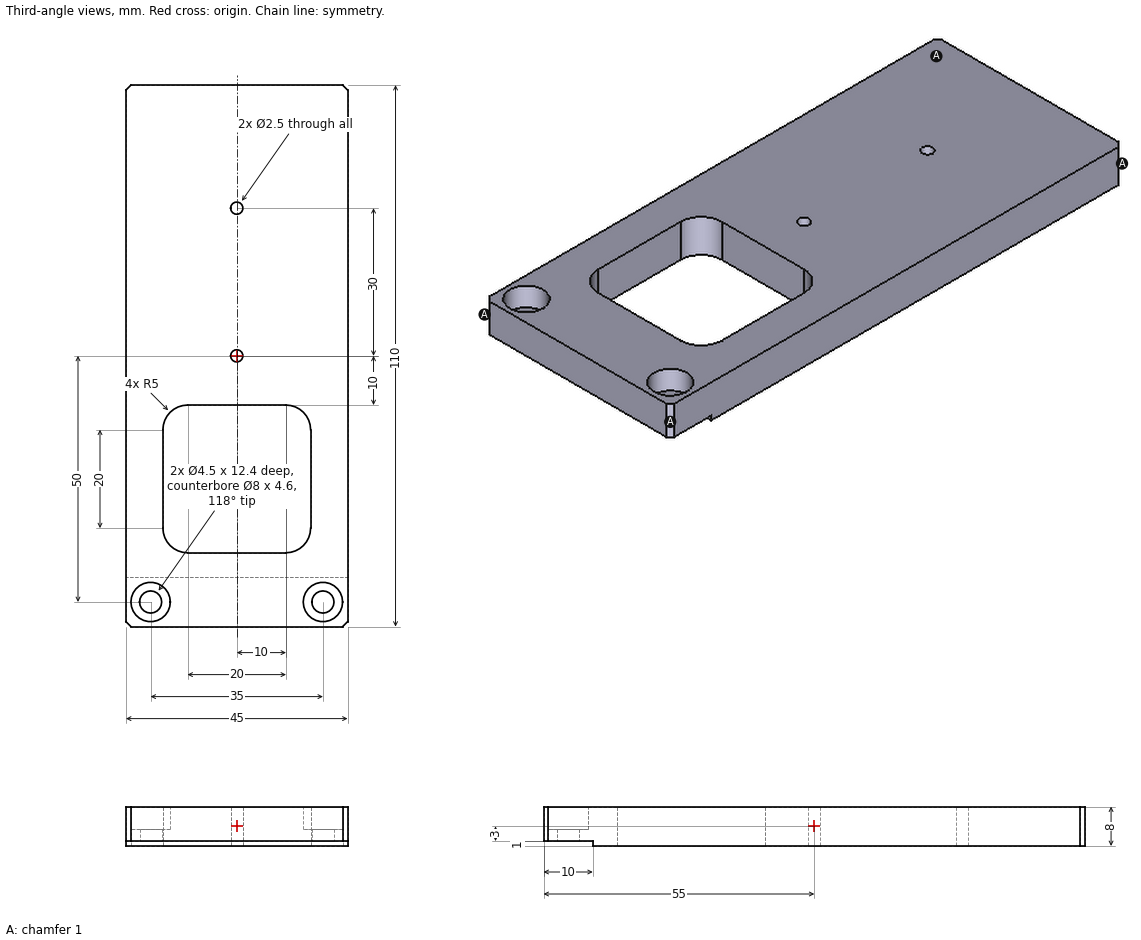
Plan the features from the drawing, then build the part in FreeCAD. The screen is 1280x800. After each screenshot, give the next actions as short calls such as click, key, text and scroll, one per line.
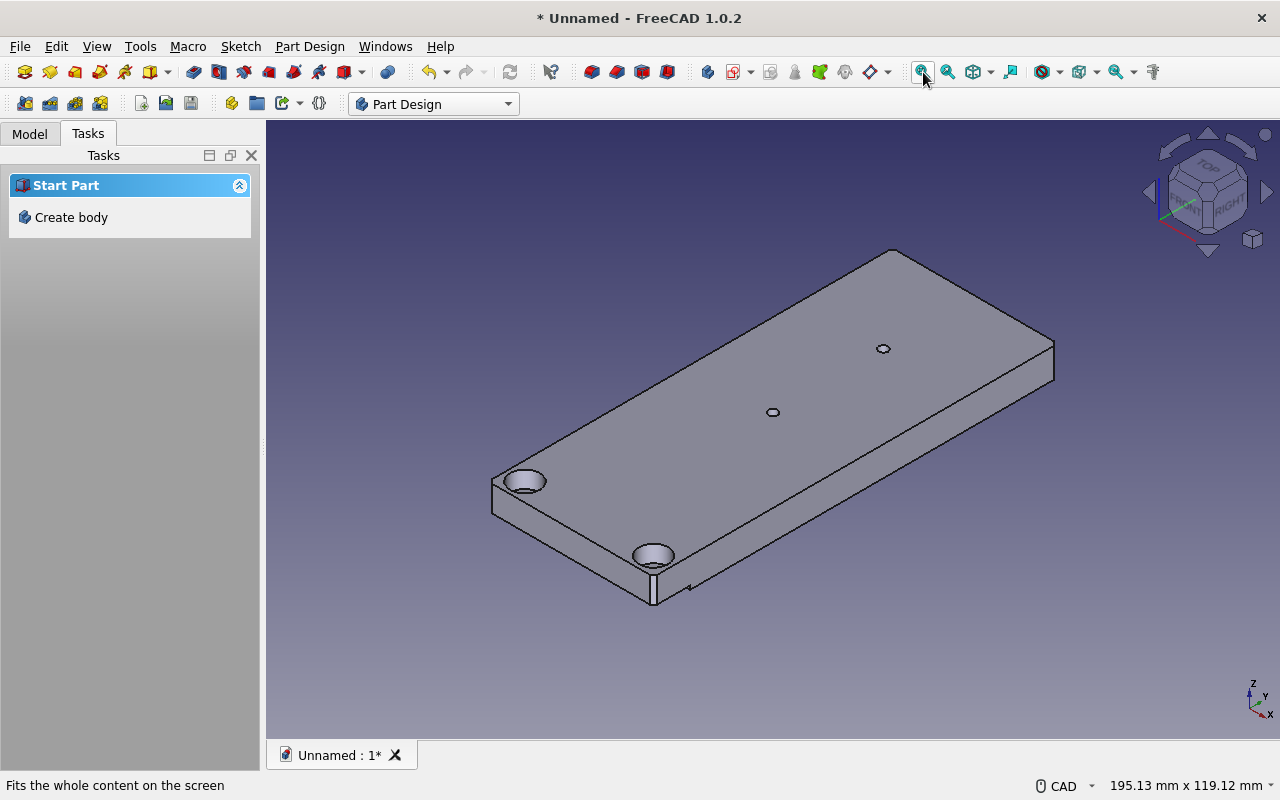
click(658, 478)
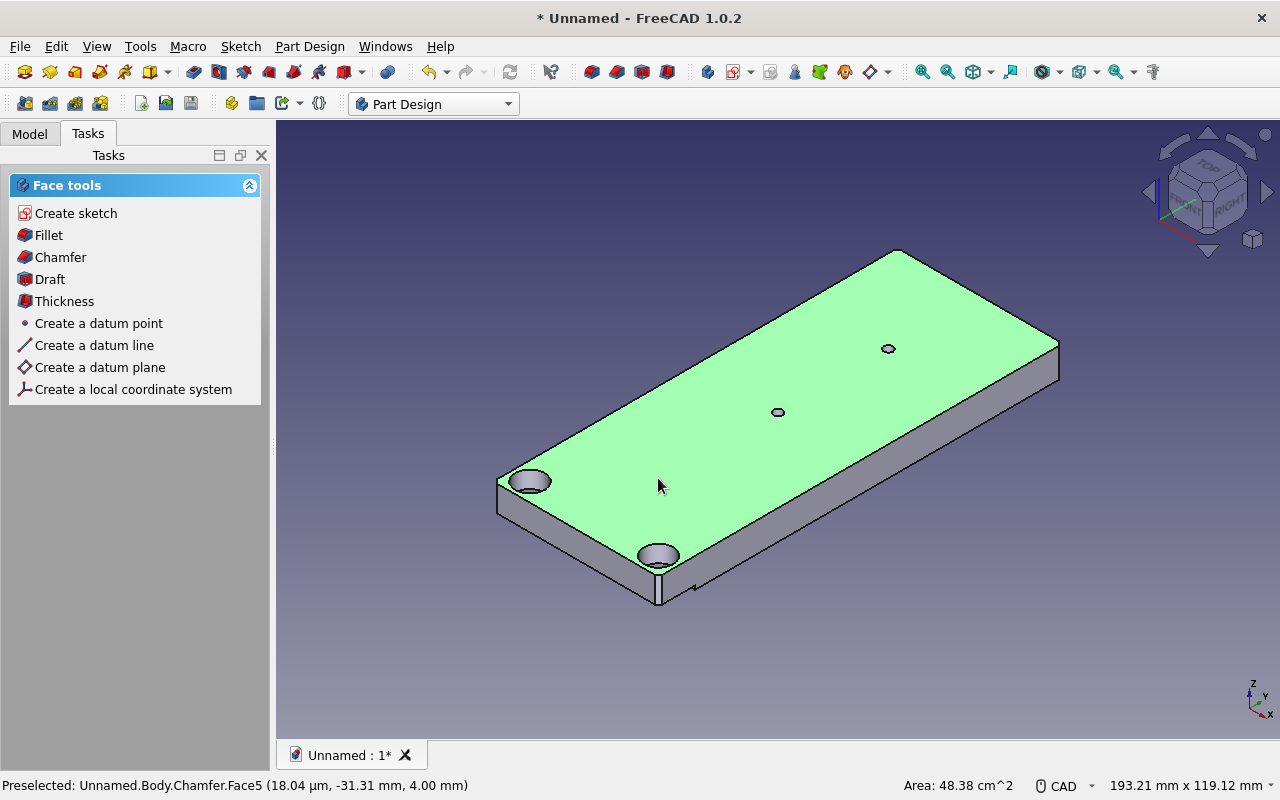
click(732, 72)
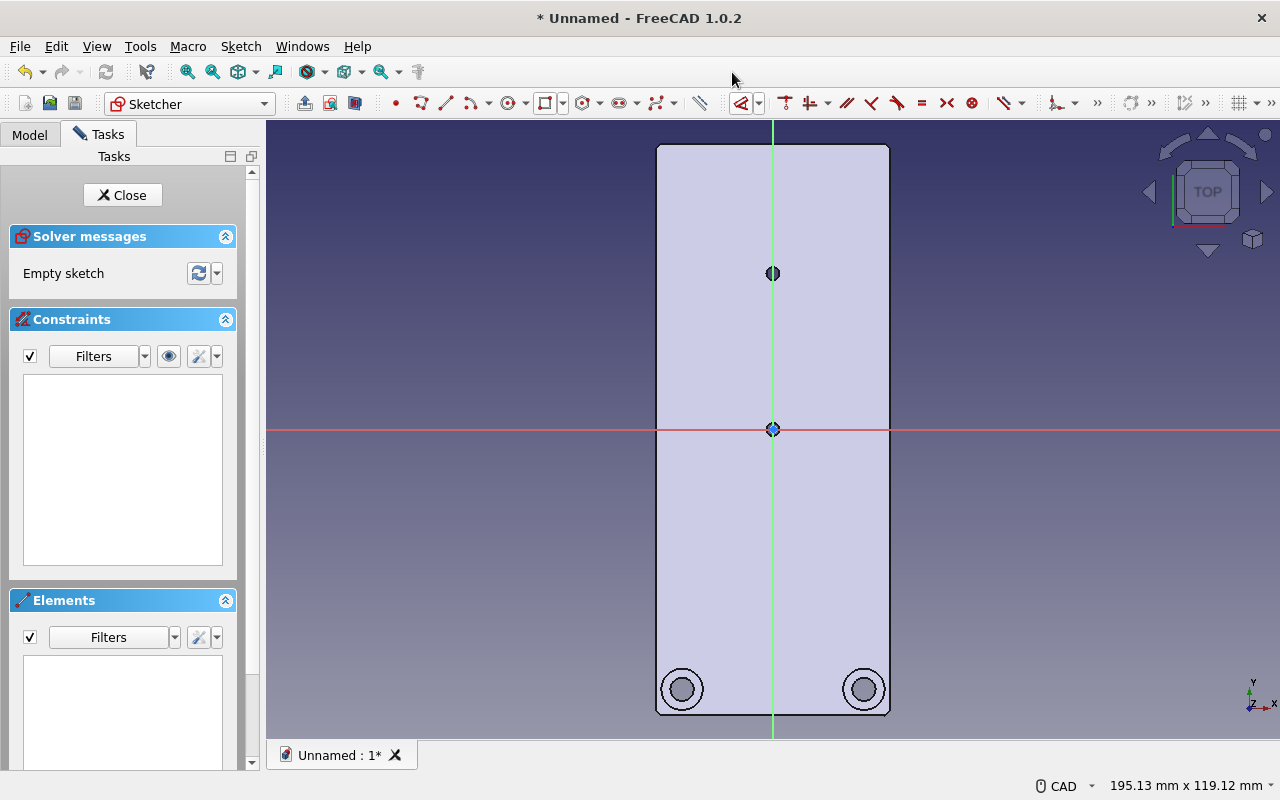
scroll(856, 660, up, 3)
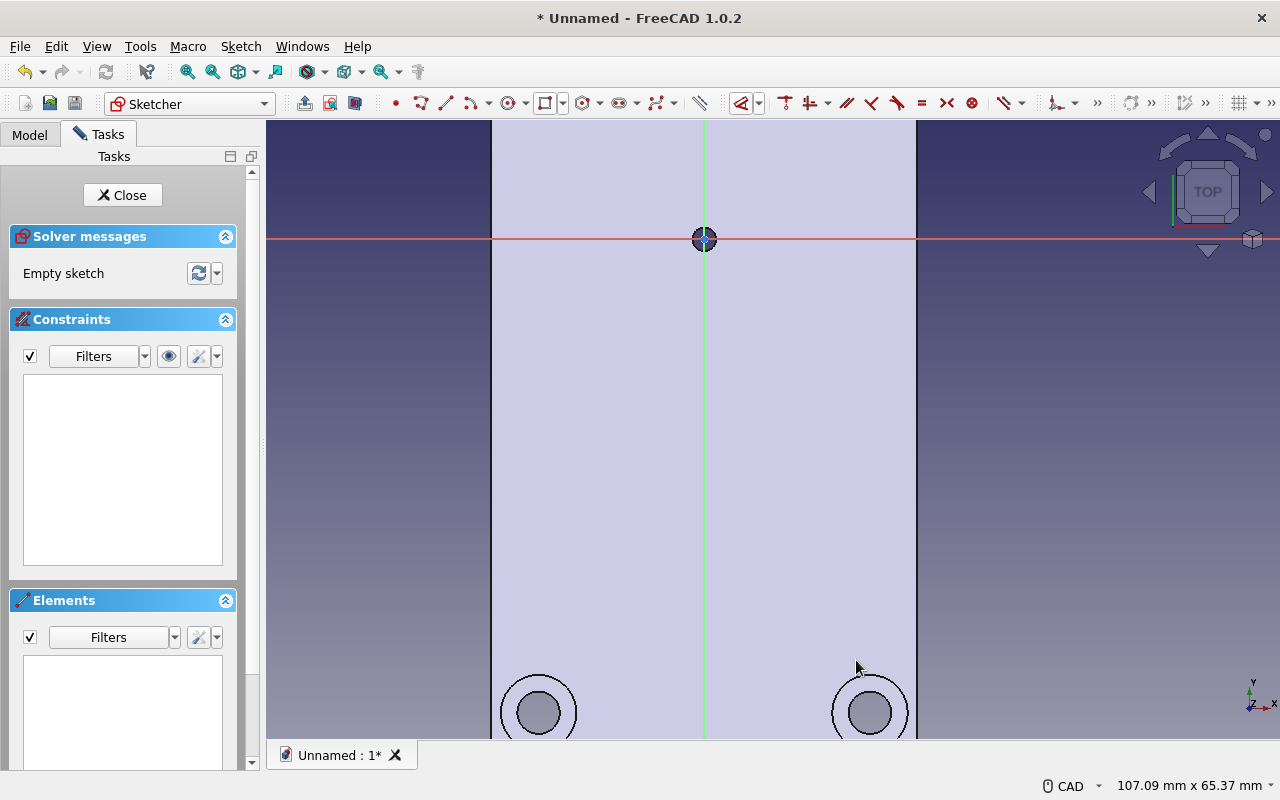
click(446, 104)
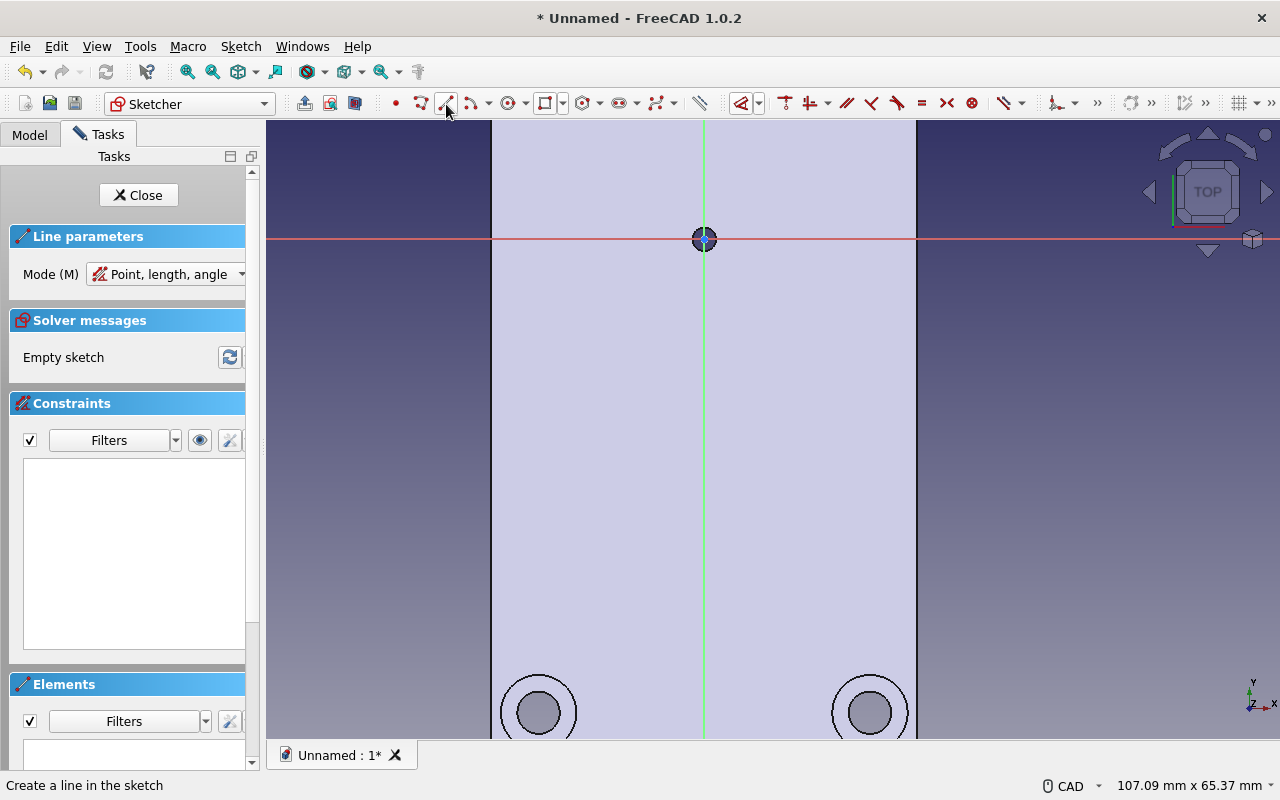
click(799, 334)
click(610, 334)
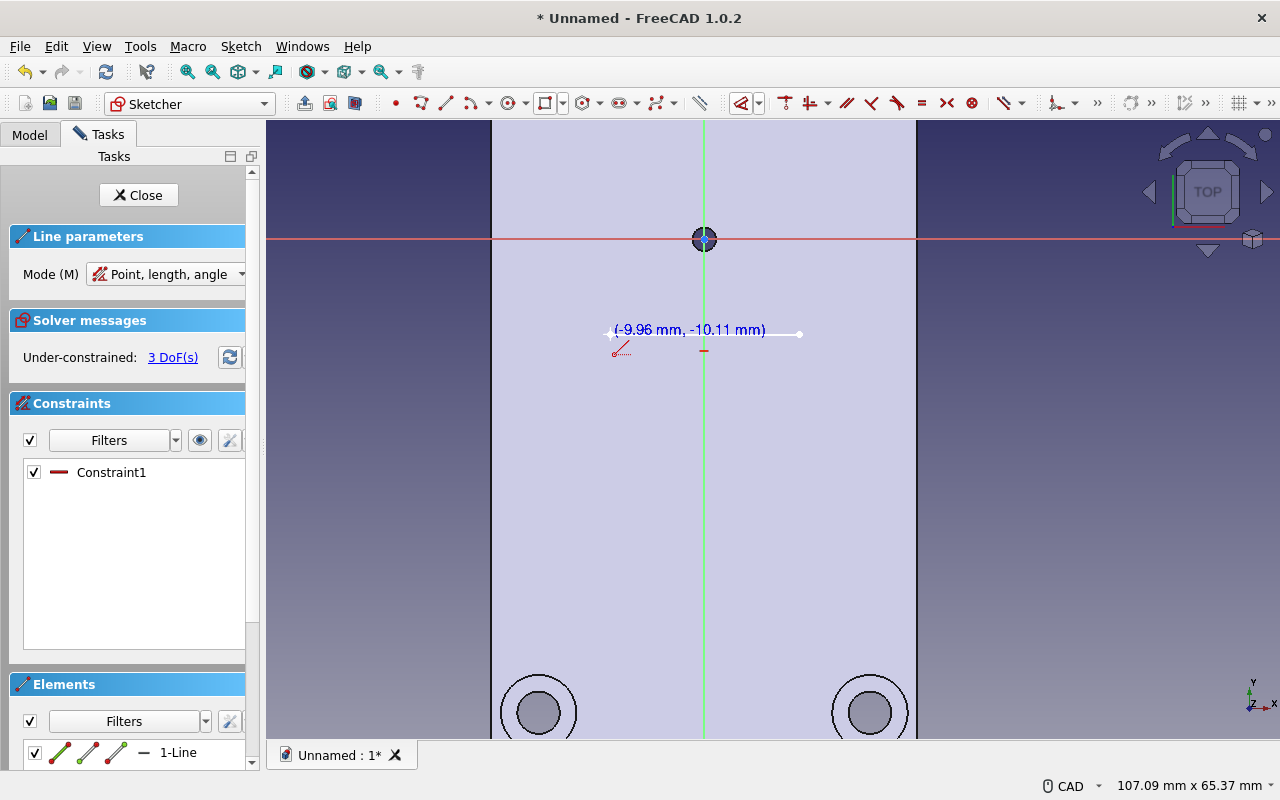
click(562, 381)
click(562, 571)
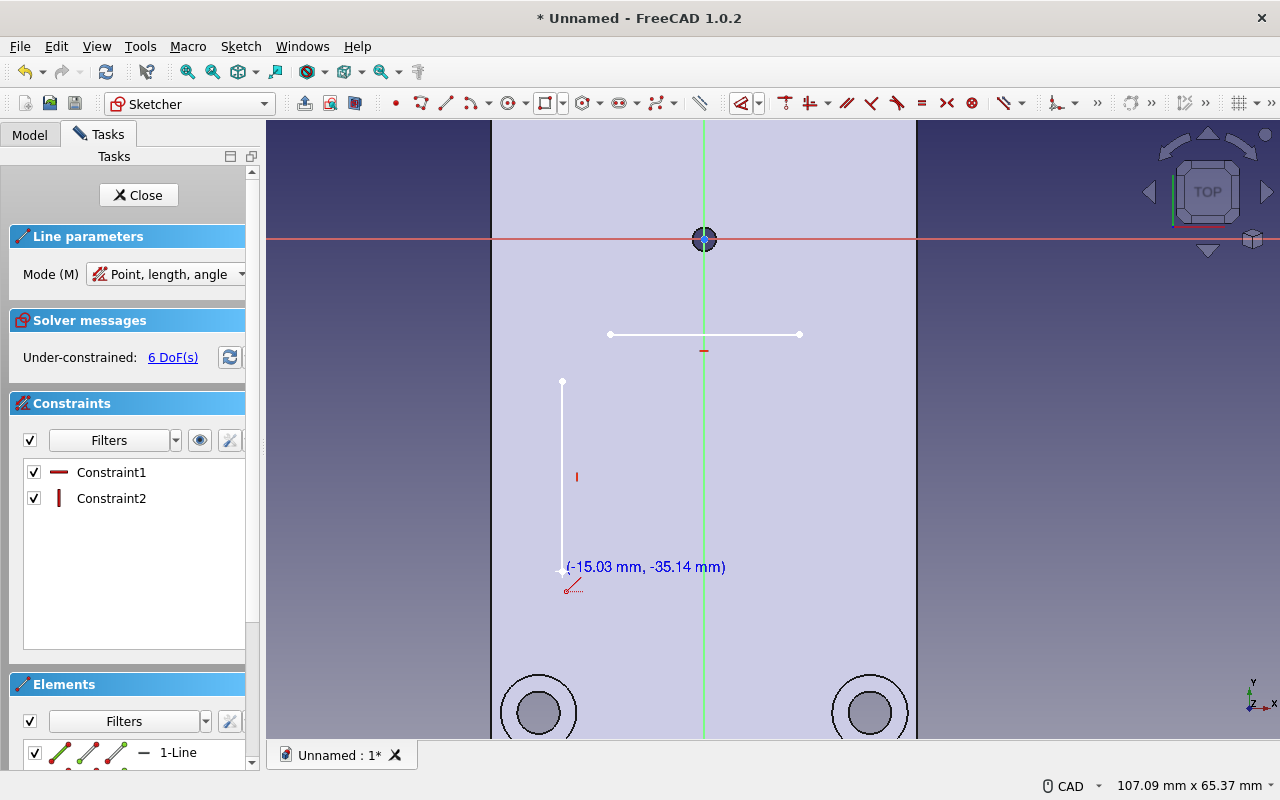
click(610, 618)
click(799, 618)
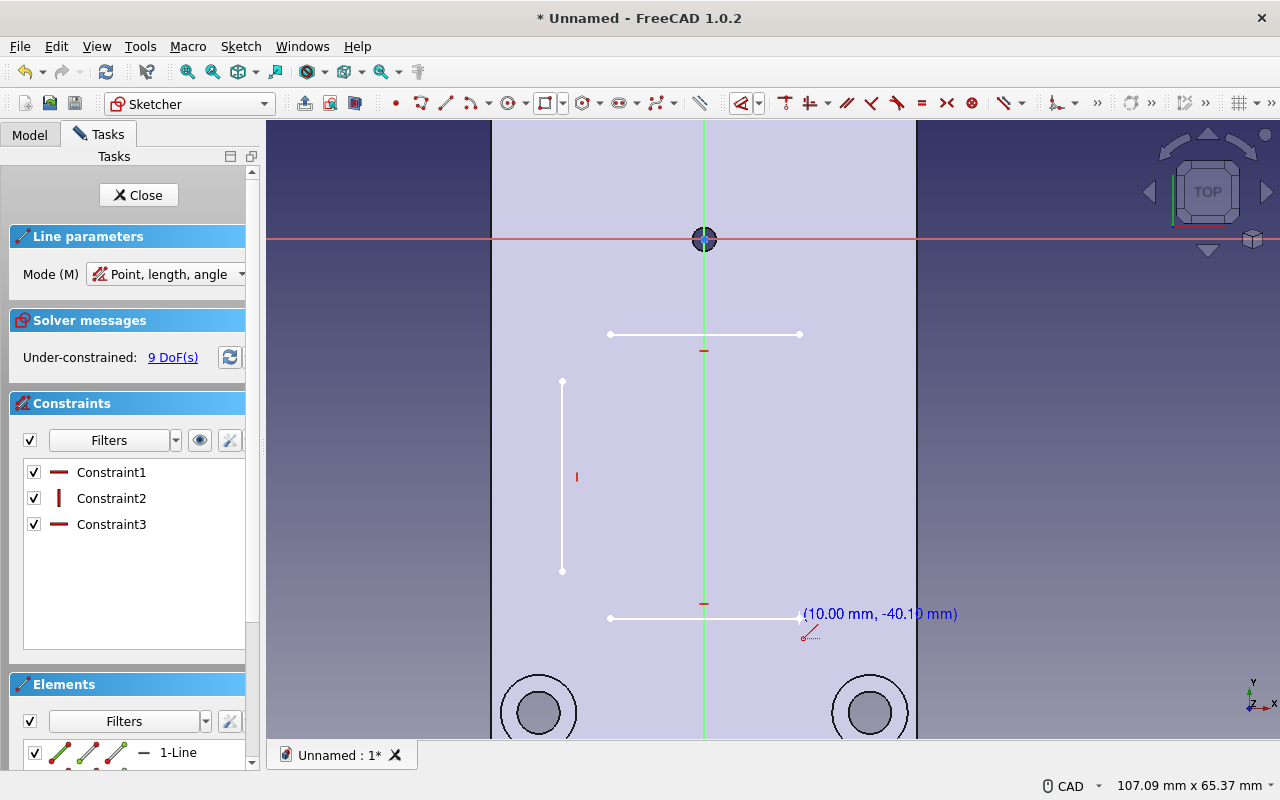
click(846, 571)
click(846, 381)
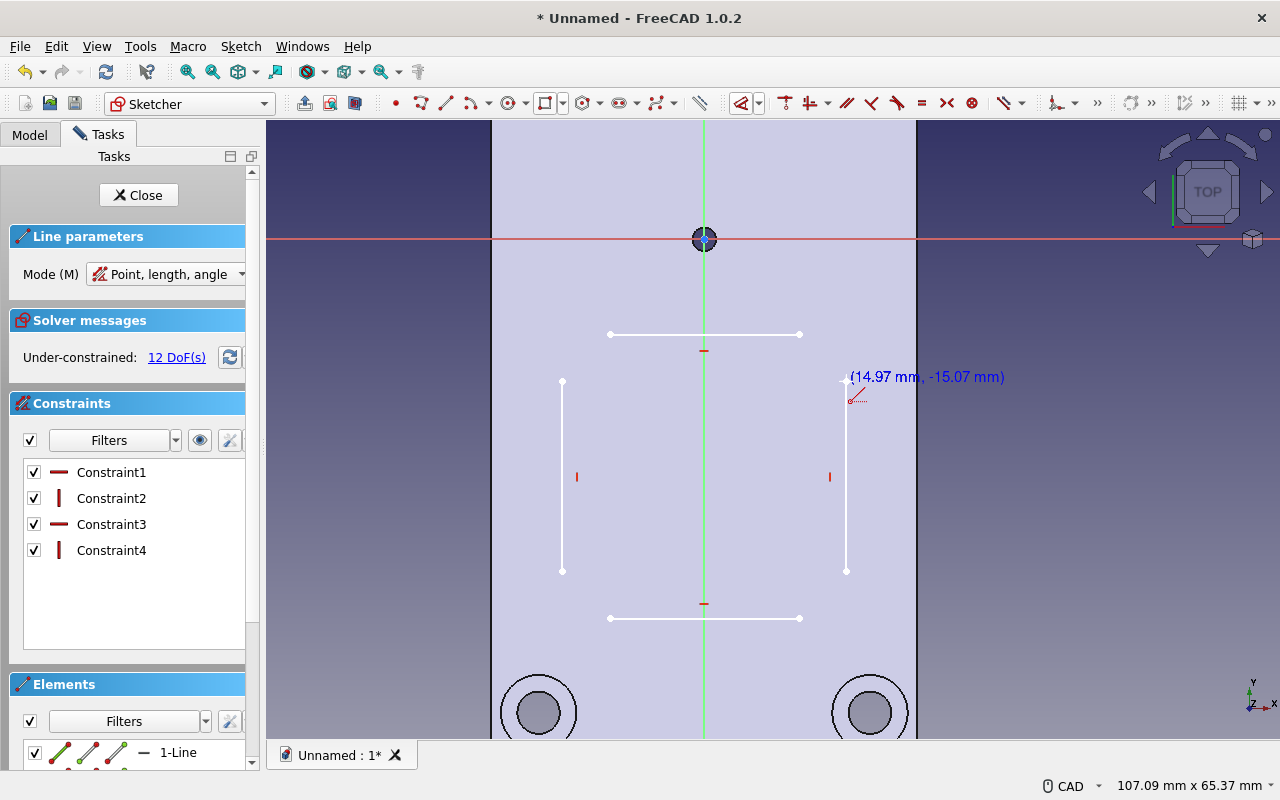
key(g)
key(3)
key(a)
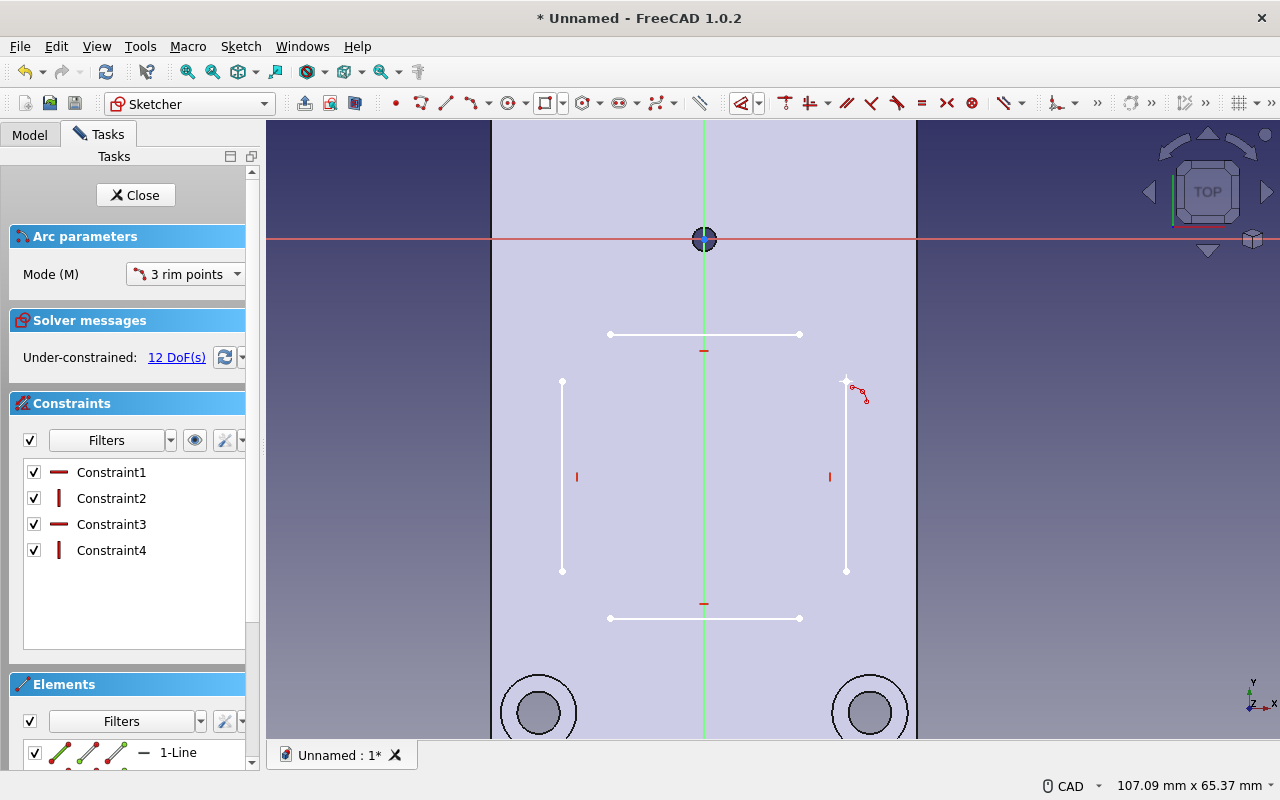
click(610, 335)
click(562, 382)
click(576, 348)